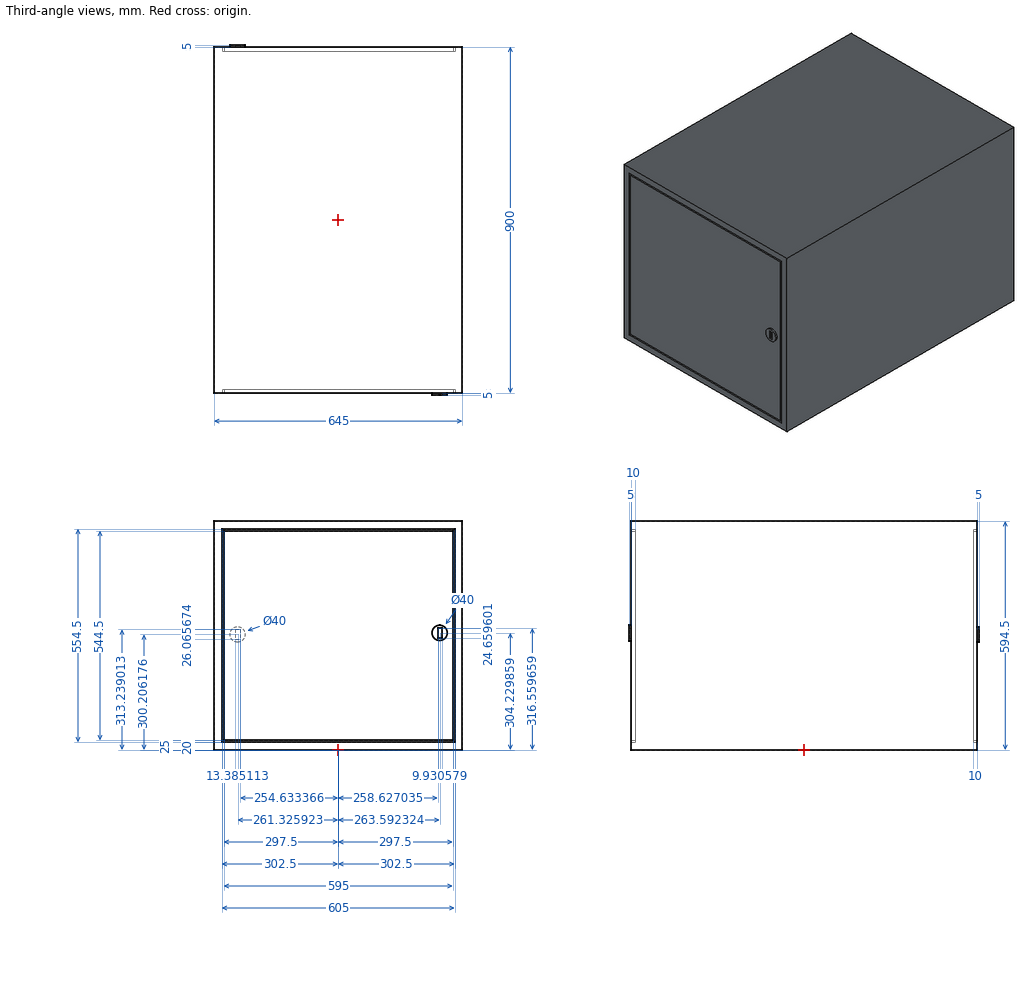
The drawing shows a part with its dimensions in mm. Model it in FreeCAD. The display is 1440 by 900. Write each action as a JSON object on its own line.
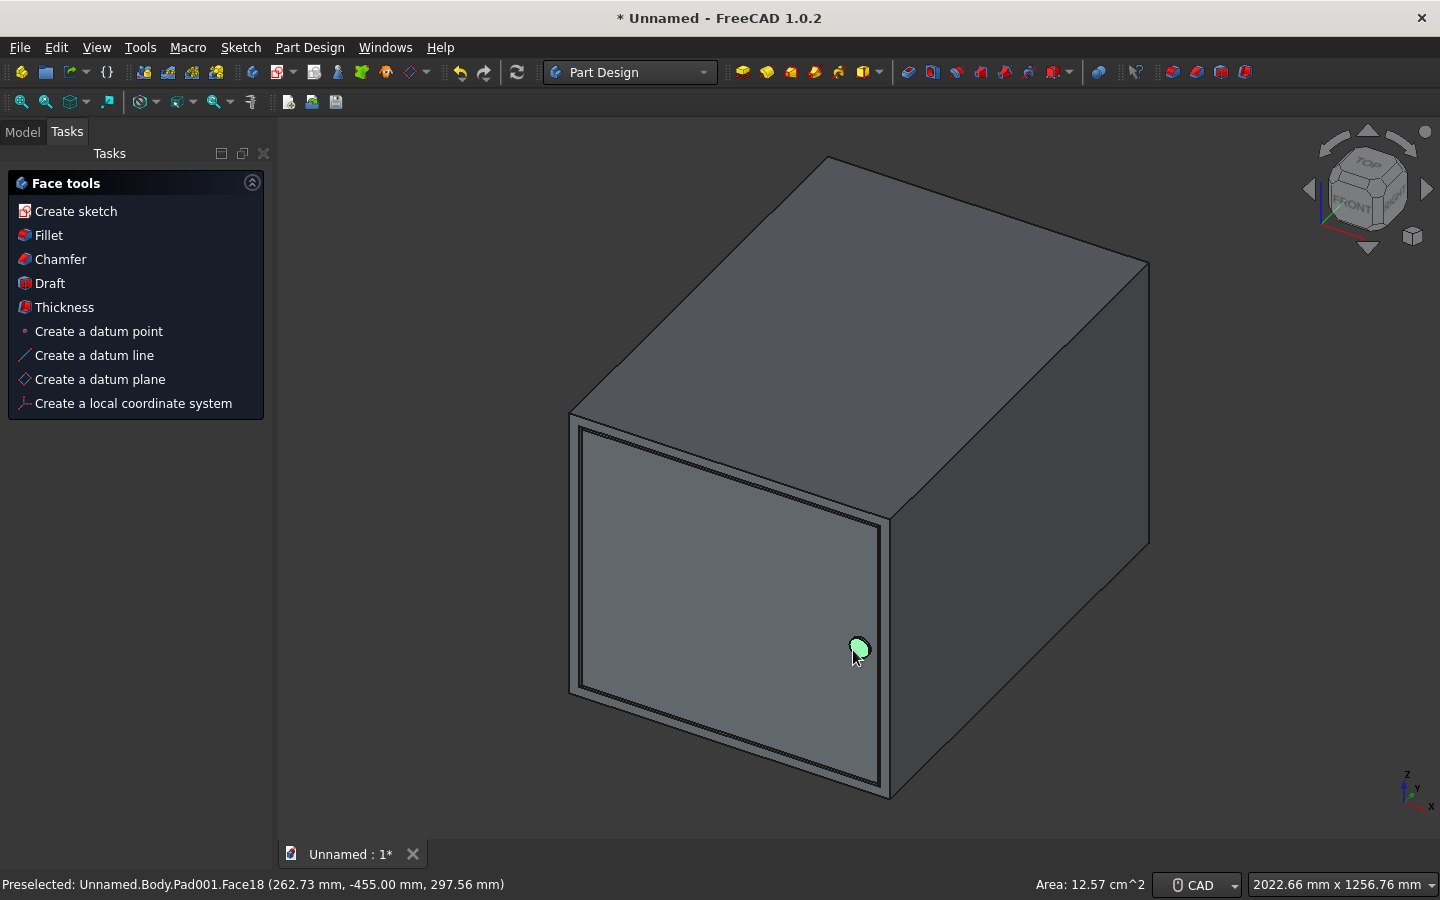
{"action": "left_click", "coordinate": [278, 72]}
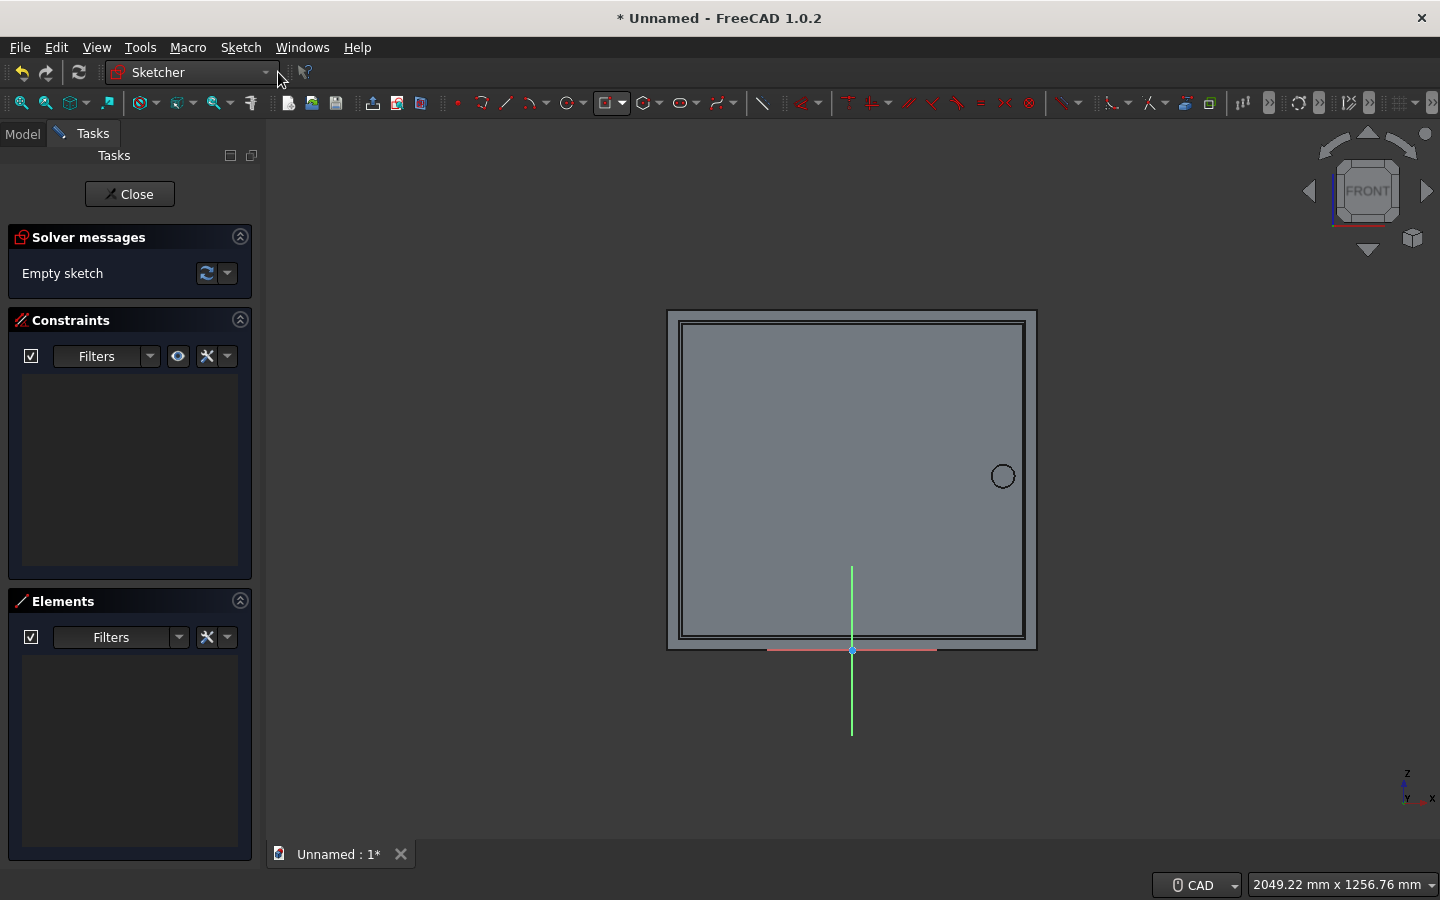
{"action": "scroll", "coordinate": [1015, 476], "scroll_direction": "up", "scroll_amount": 15}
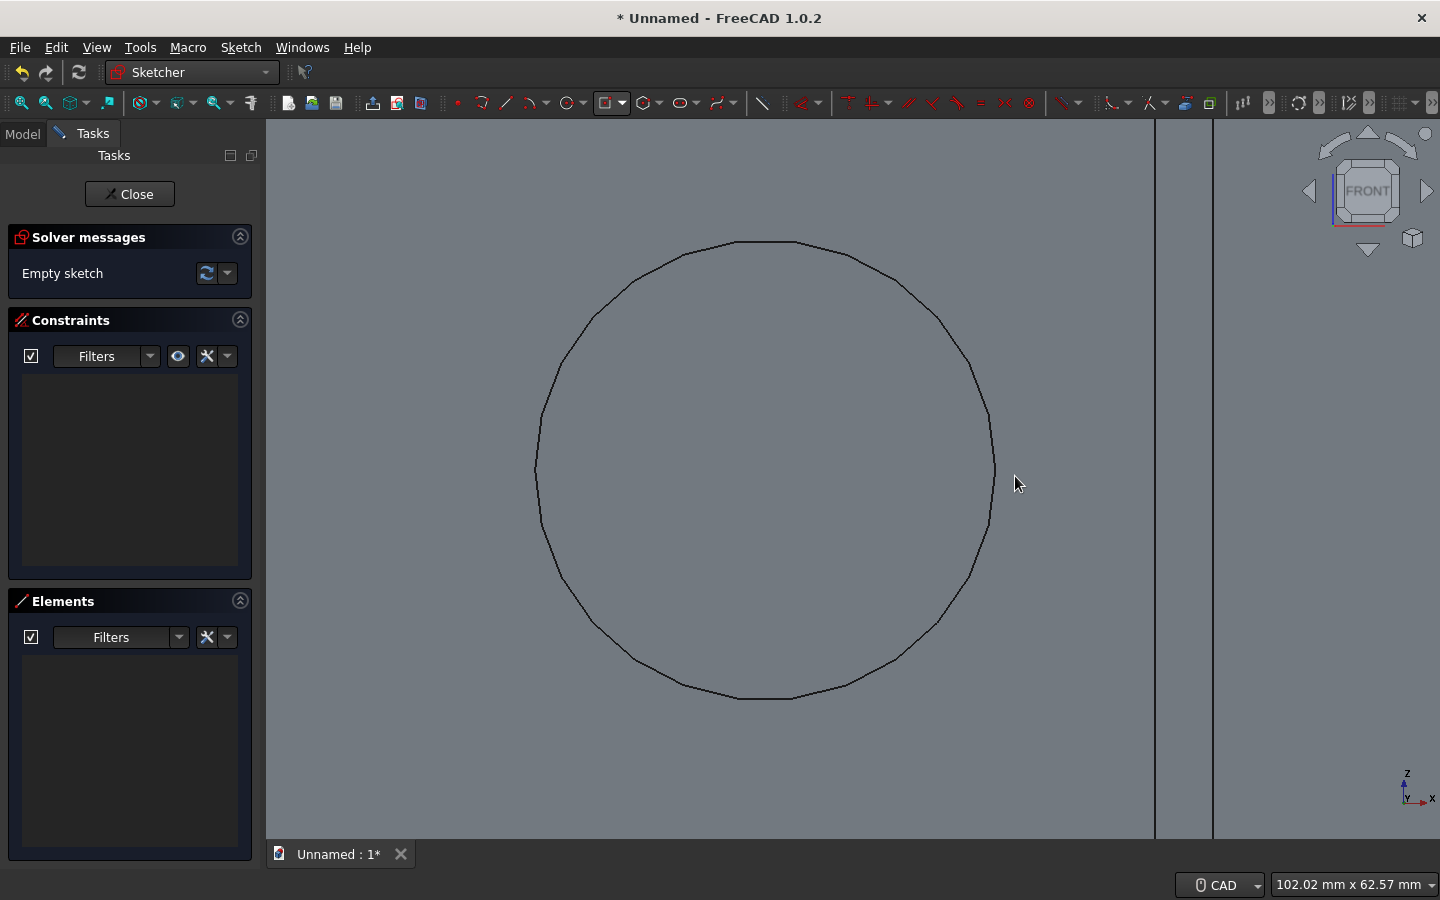
{"action": "scroll", "coordinate": [742, 459], "scroll_direction": "up", "scroll_amount": 3}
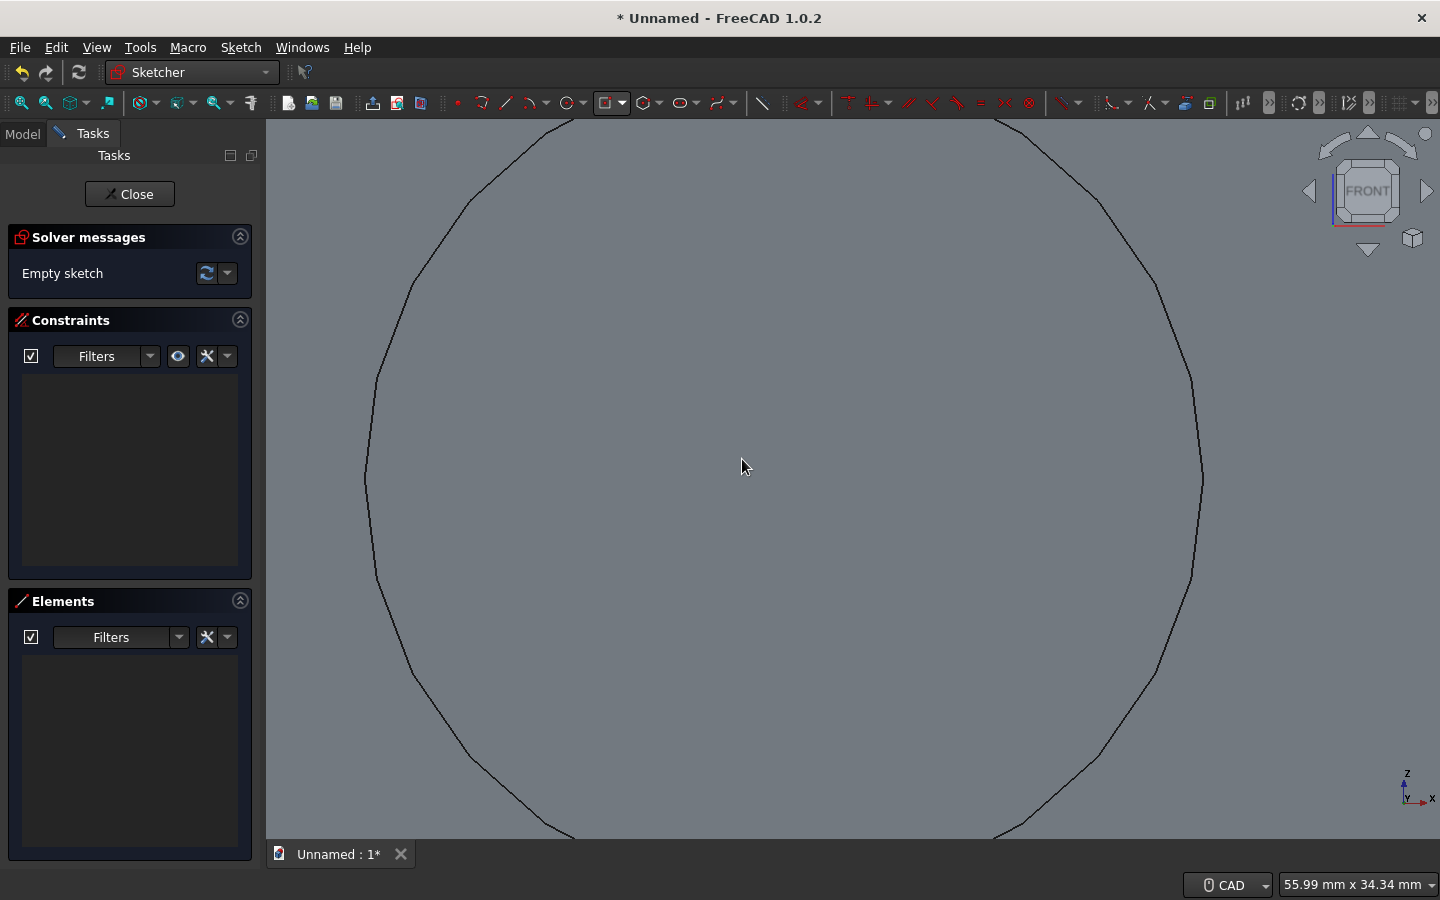
{"action": "key", "text": "g r"}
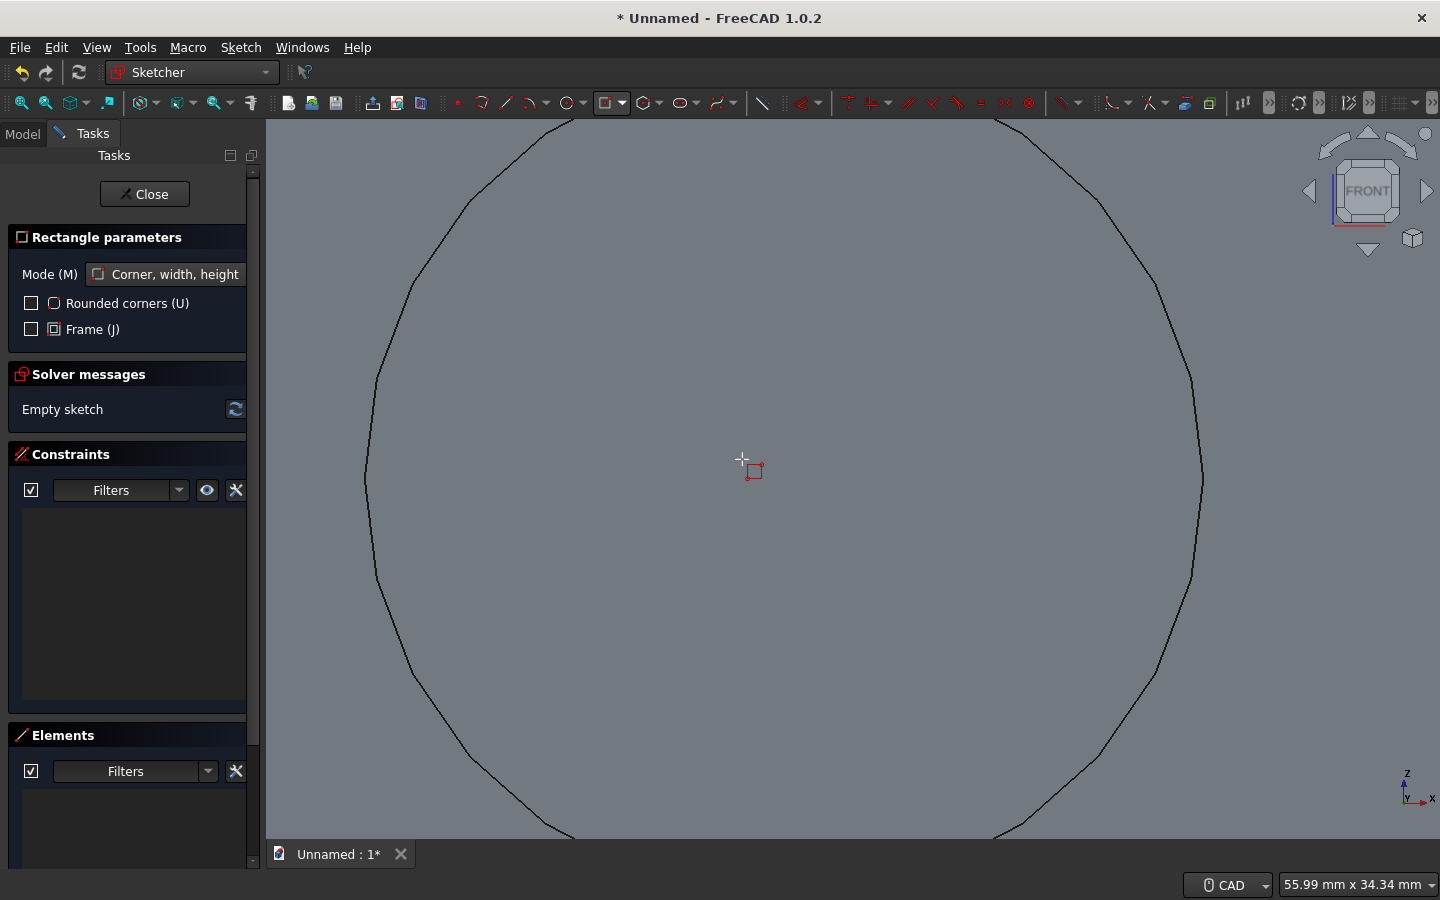
{"action": "left_click", "coordinate": [680, 220]}
{"action": "left_click", "coordinate": [888, 737]}
{"action": "key", "text": "Escape"}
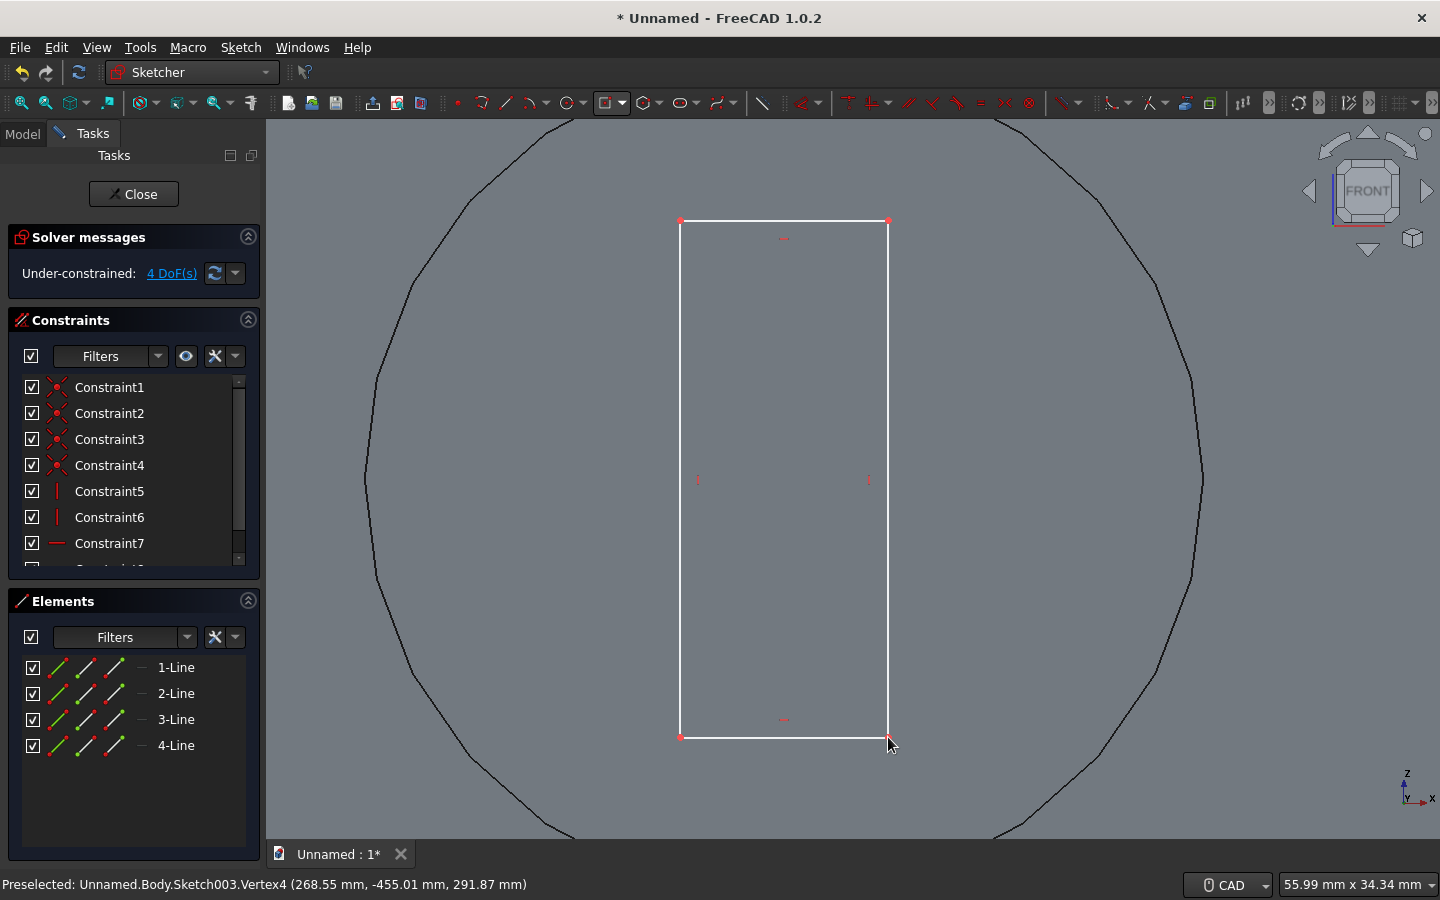
{"action": "key", "text": "d"}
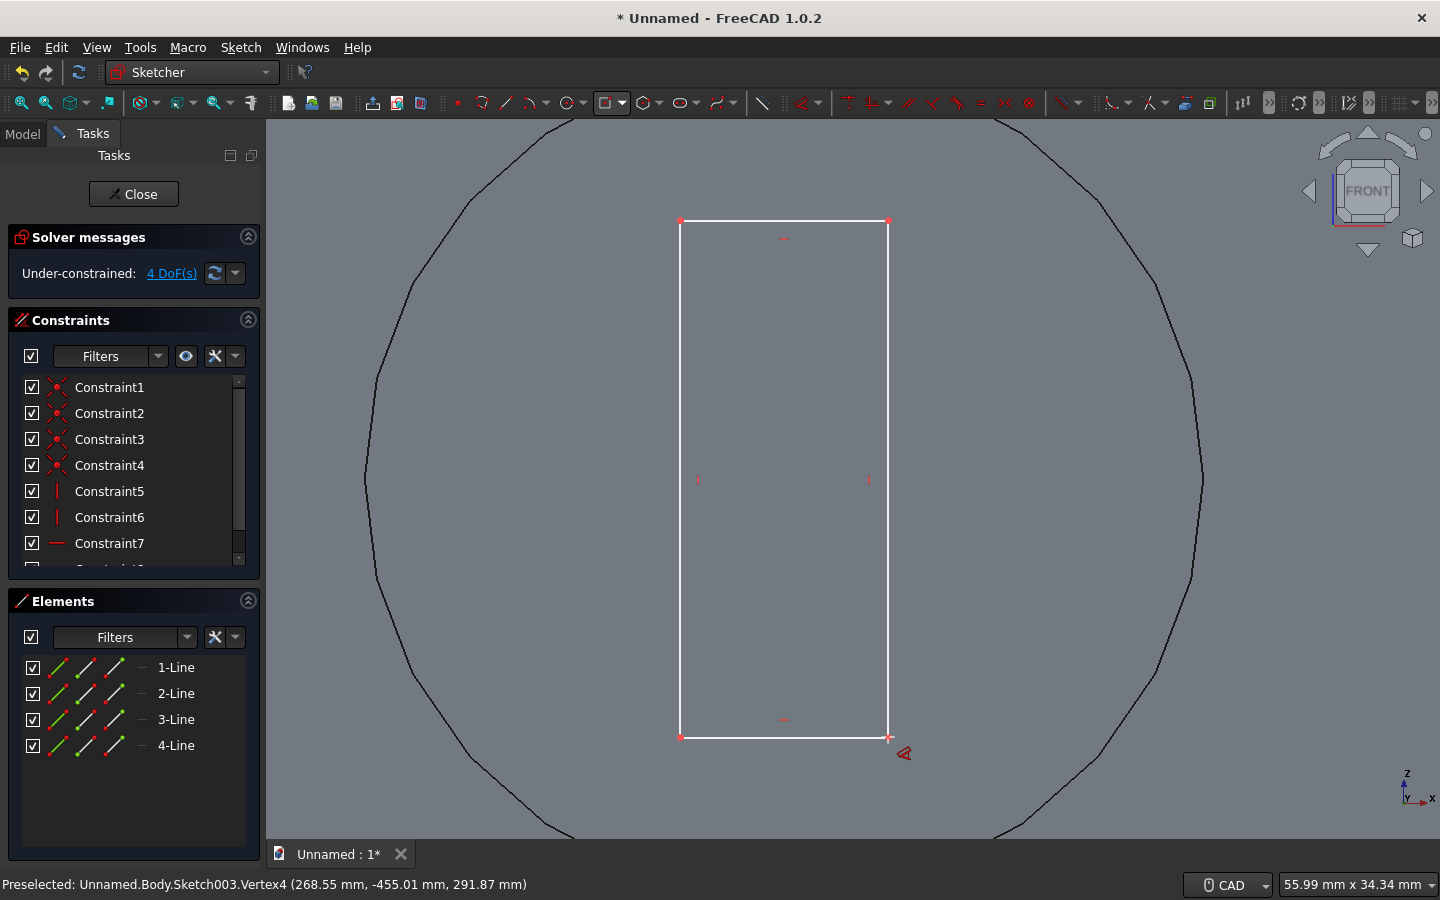
{"action": "left_click", "coordinate": [742, 738]}
{"action": "left_click", "coordinate": [784, 772]}